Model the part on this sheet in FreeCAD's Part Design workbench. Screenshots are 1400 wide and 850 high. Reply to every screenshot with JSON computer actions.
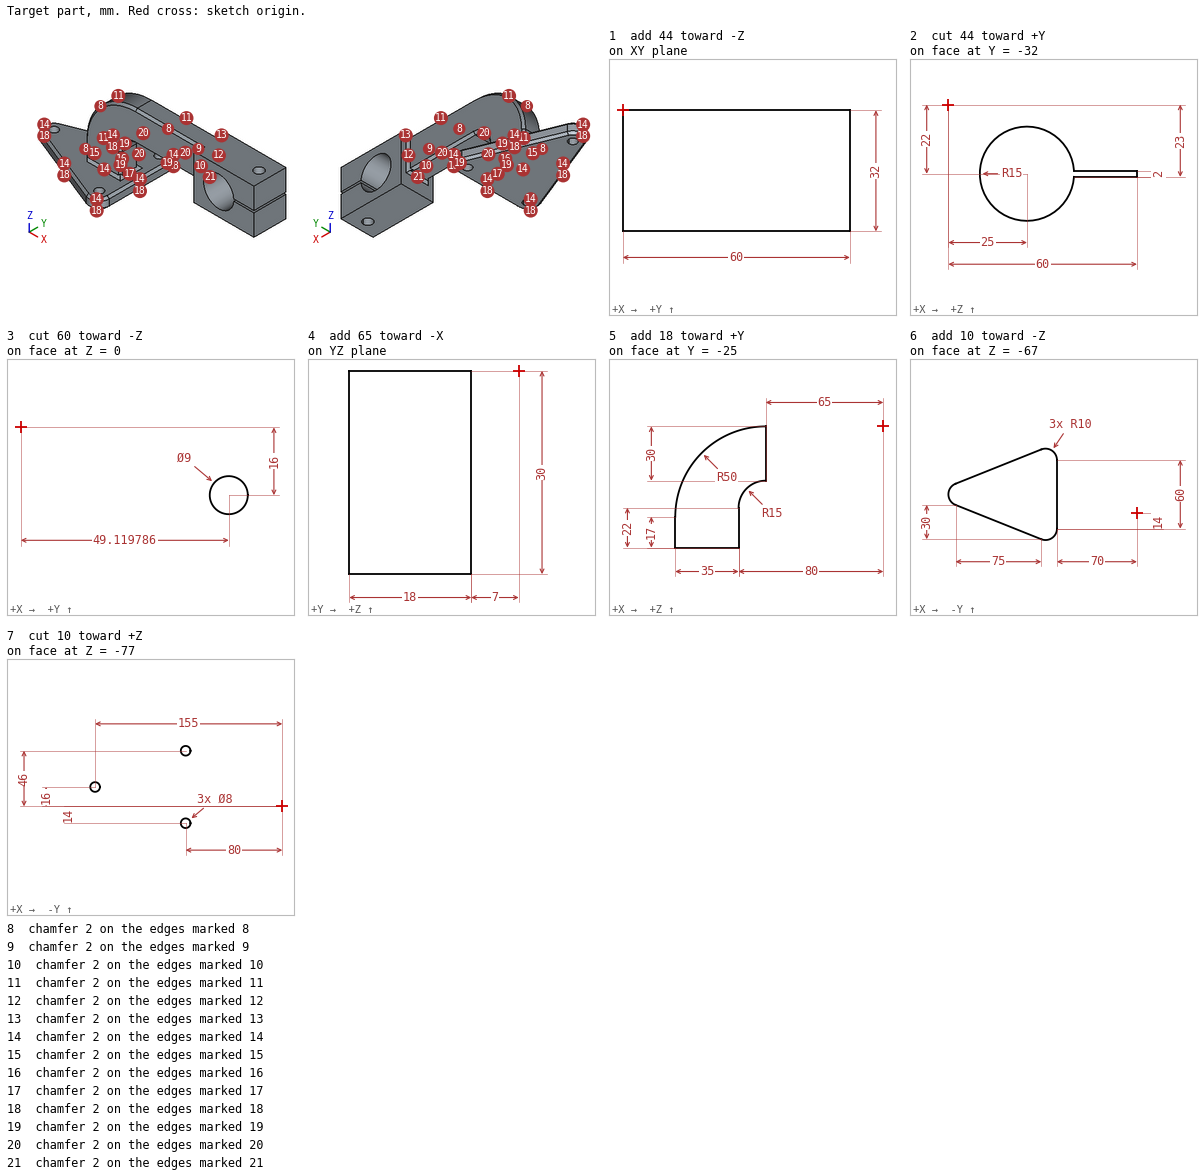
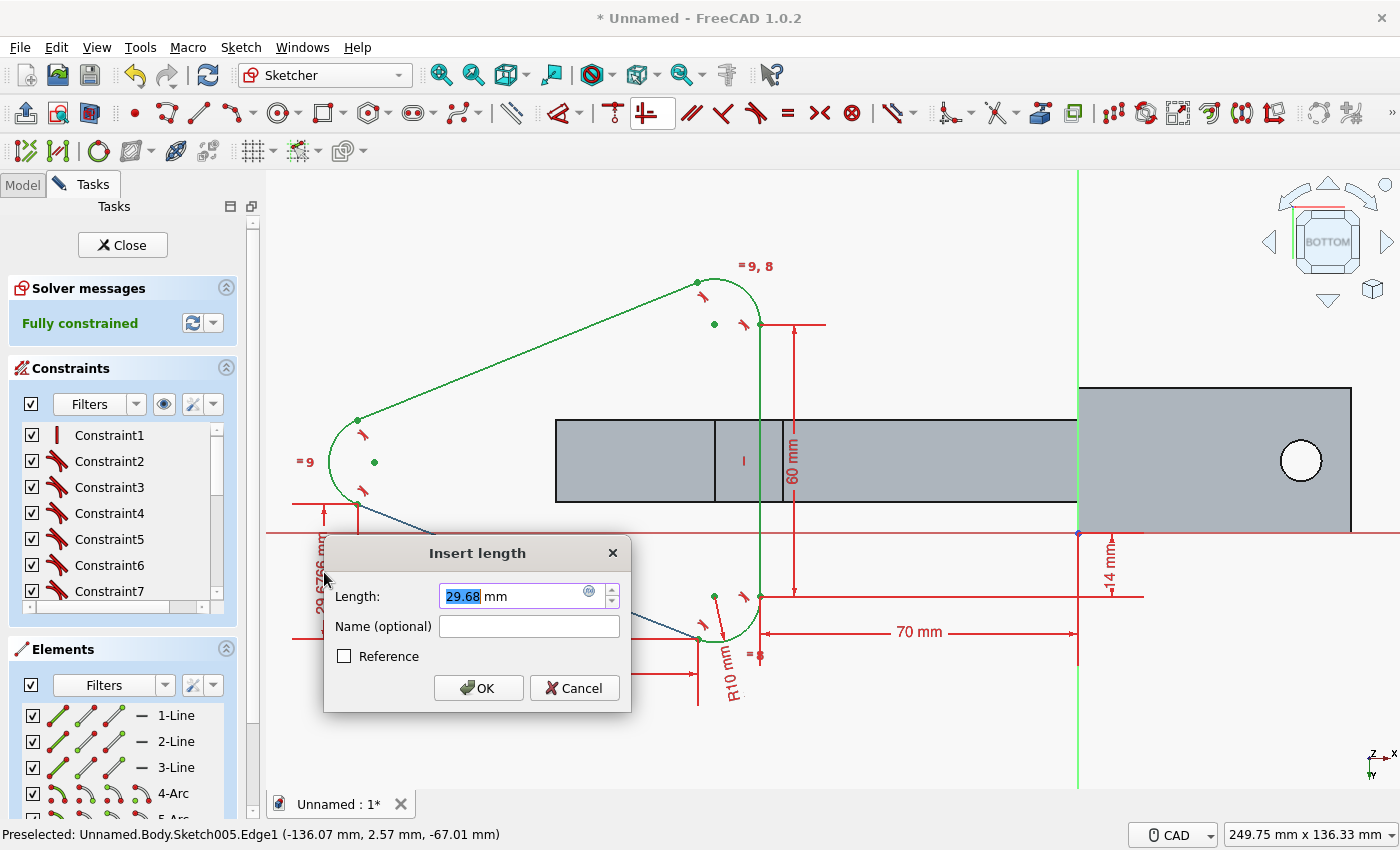
{"action": "type", "text": "30"}
{"action": "key", "text": "Return"}
{"action": "key", "text": "Escape"}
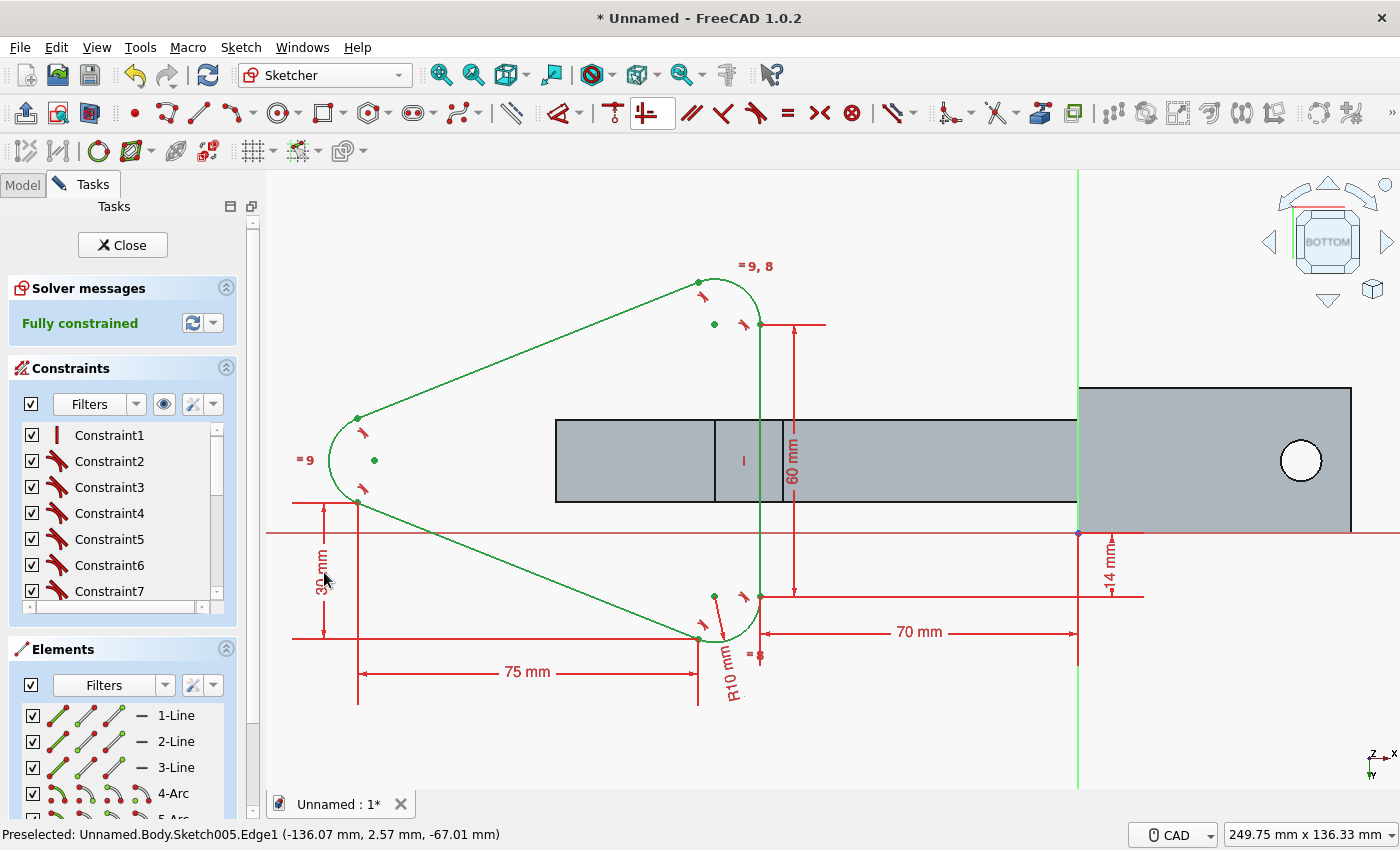
{"action": "left_click", "coordinate": [123, 245]}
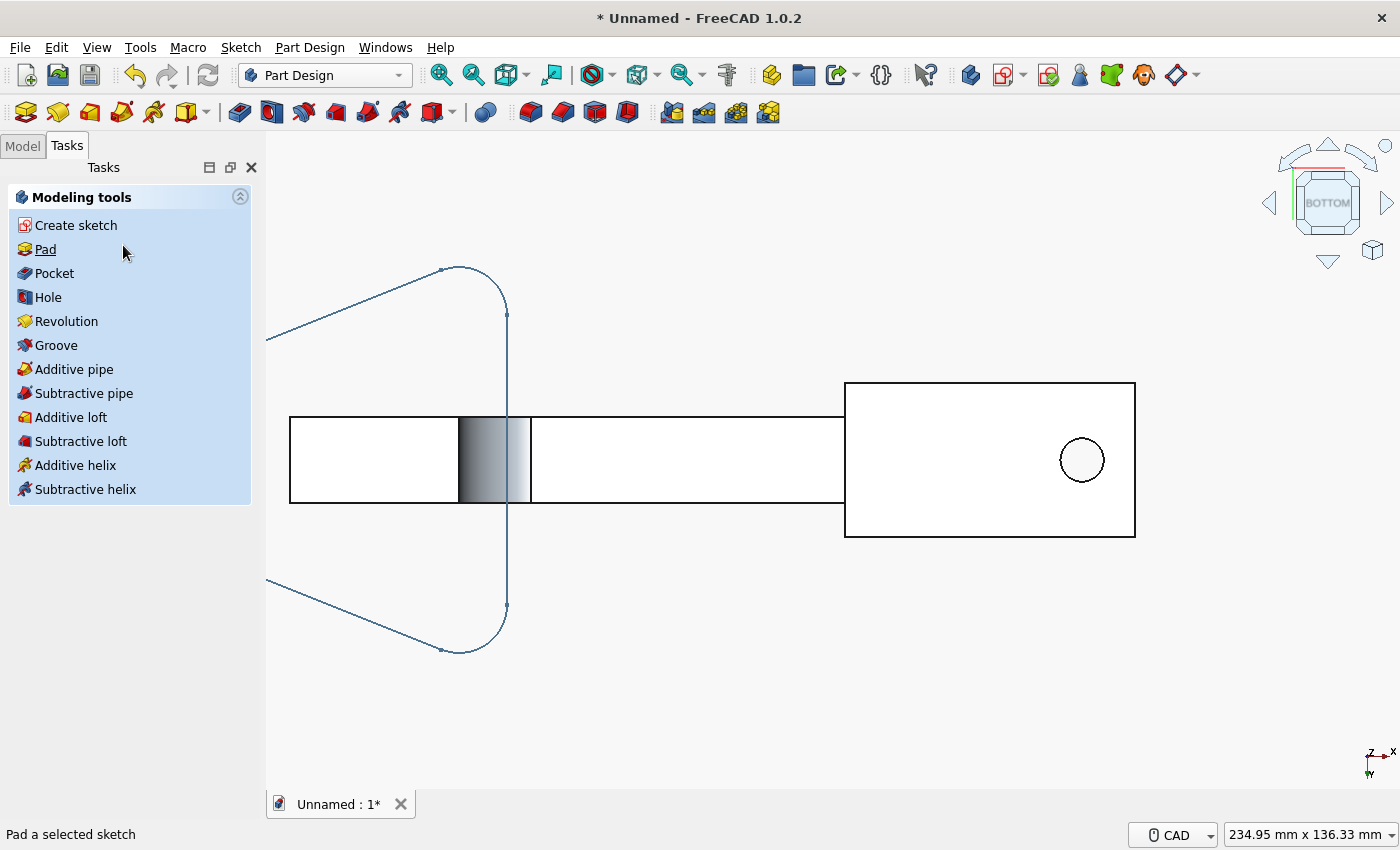
{"action": "left_click", "coordinate": [26, 112]}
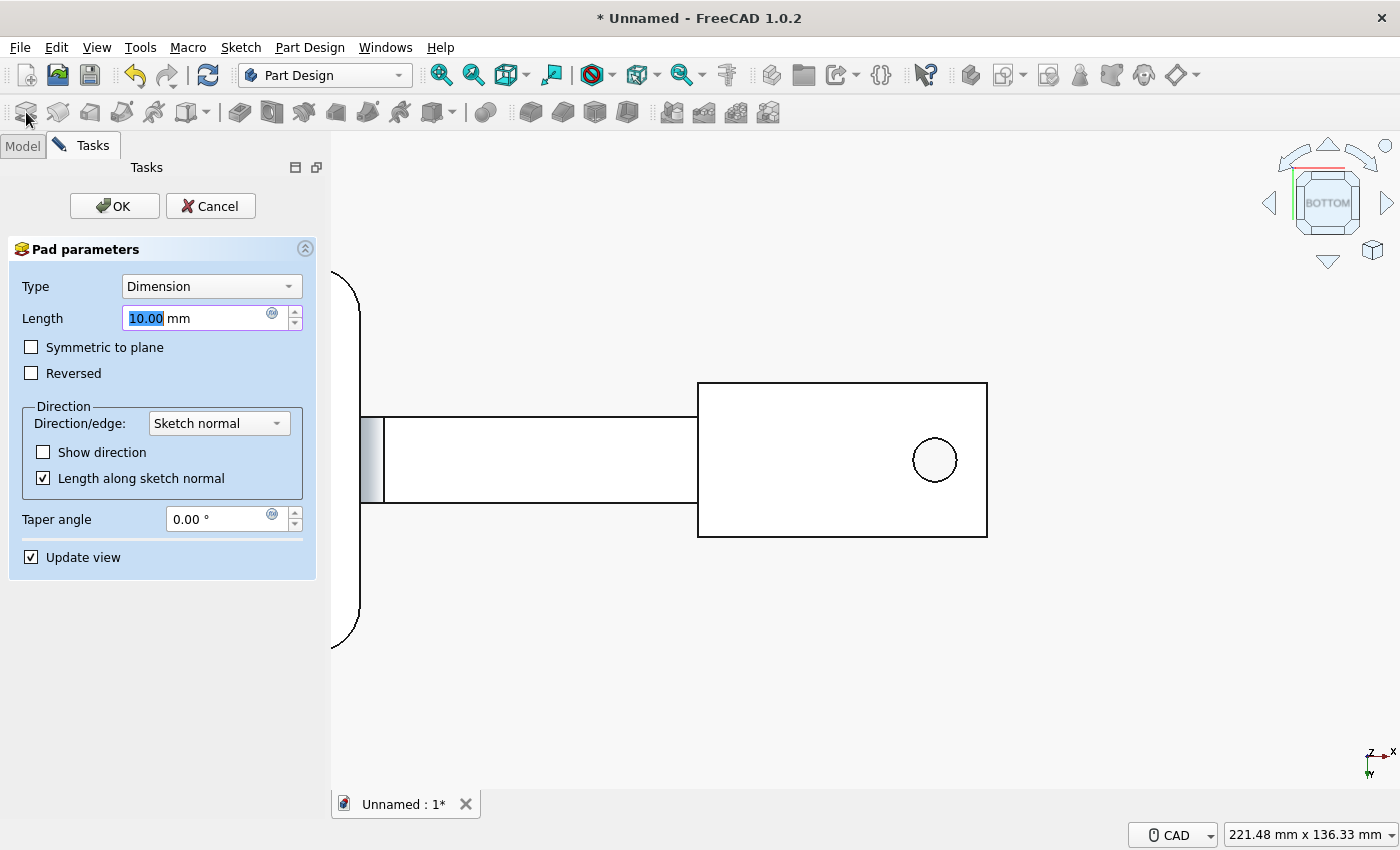
{"action": "type", "text": "10"}
{"action": "key", "text": "Tab"}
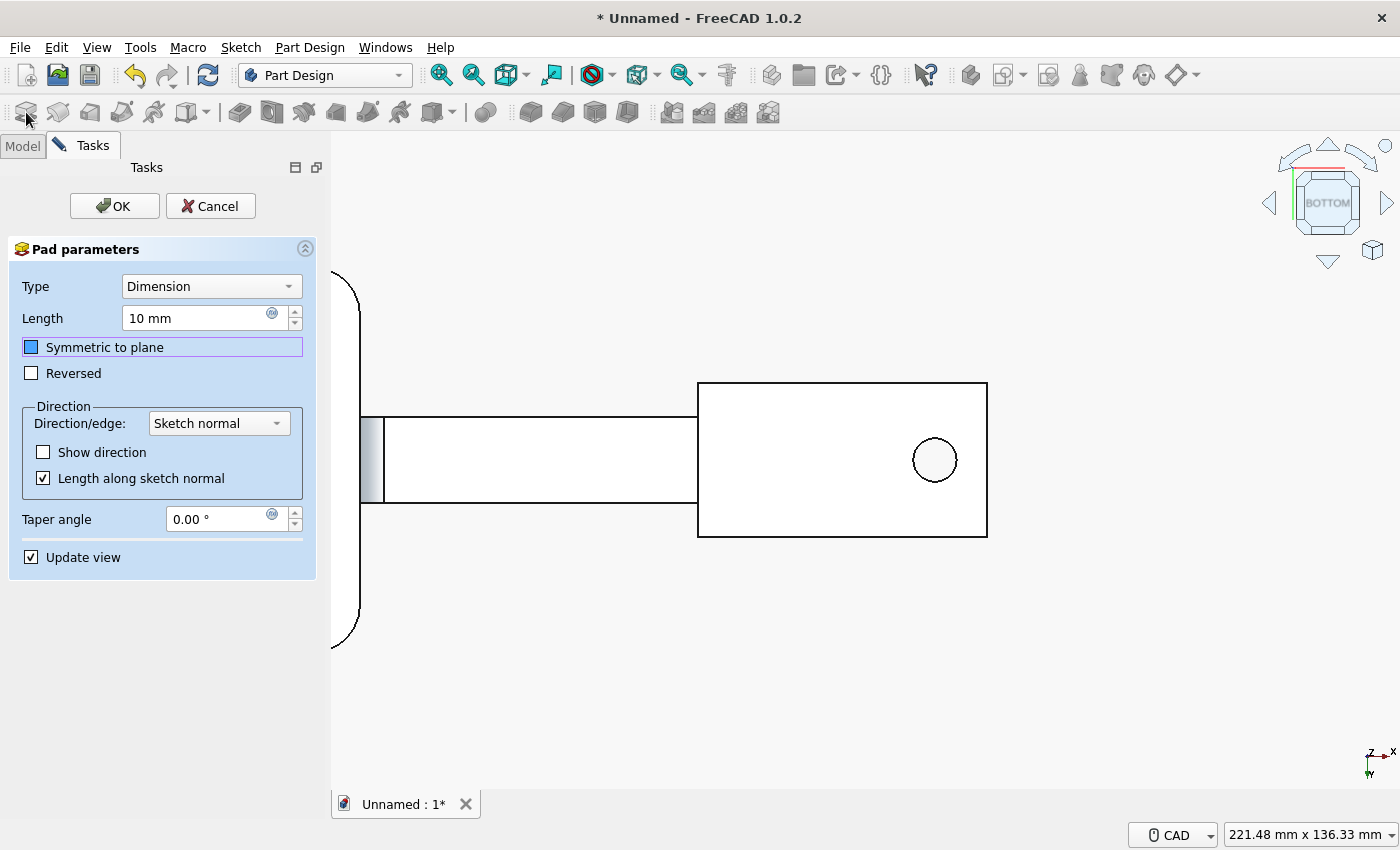
{"action": "left_click", "coordinate": [115, 206]}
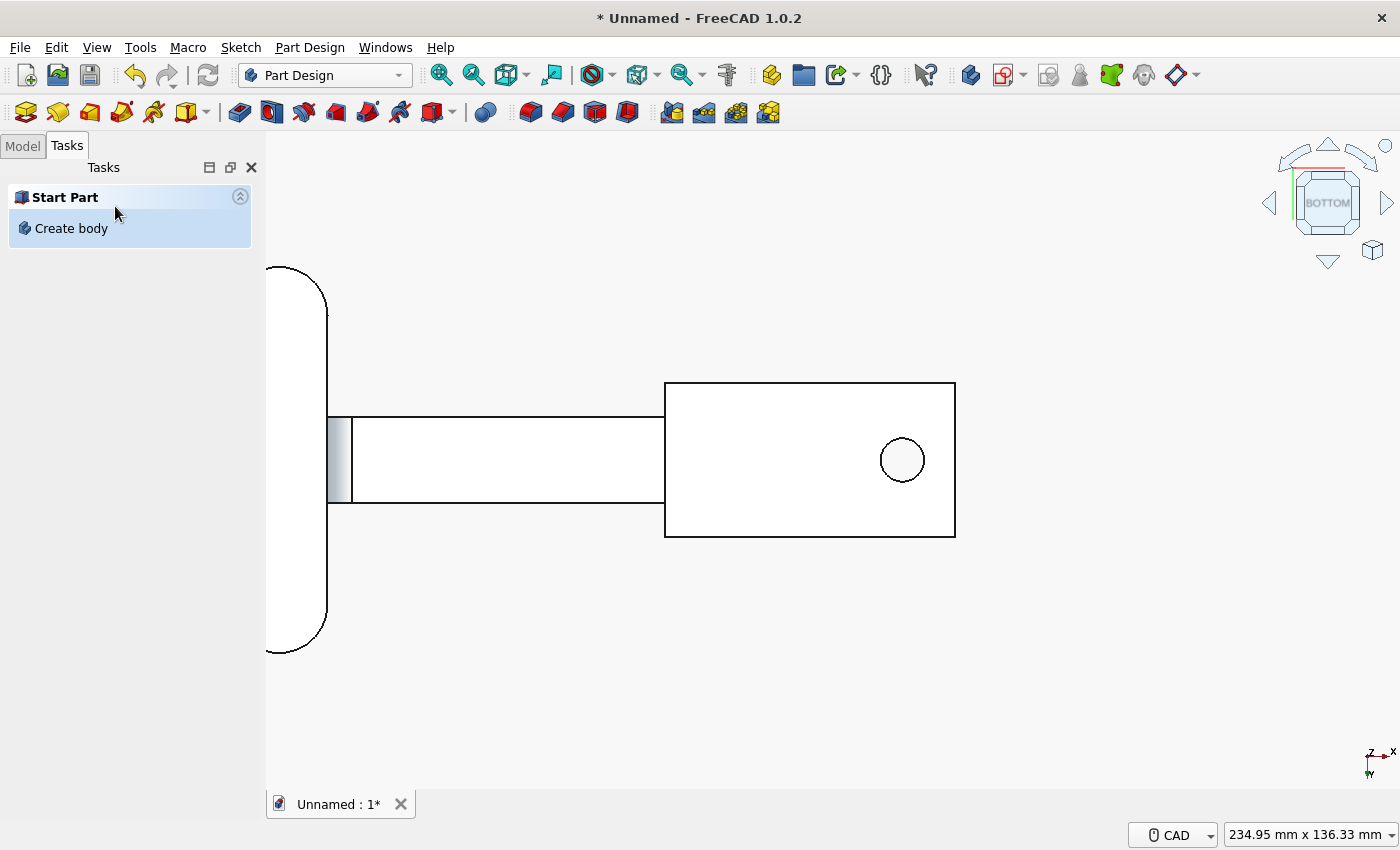
{"action": "left_click", "coordinate": [442, 76]}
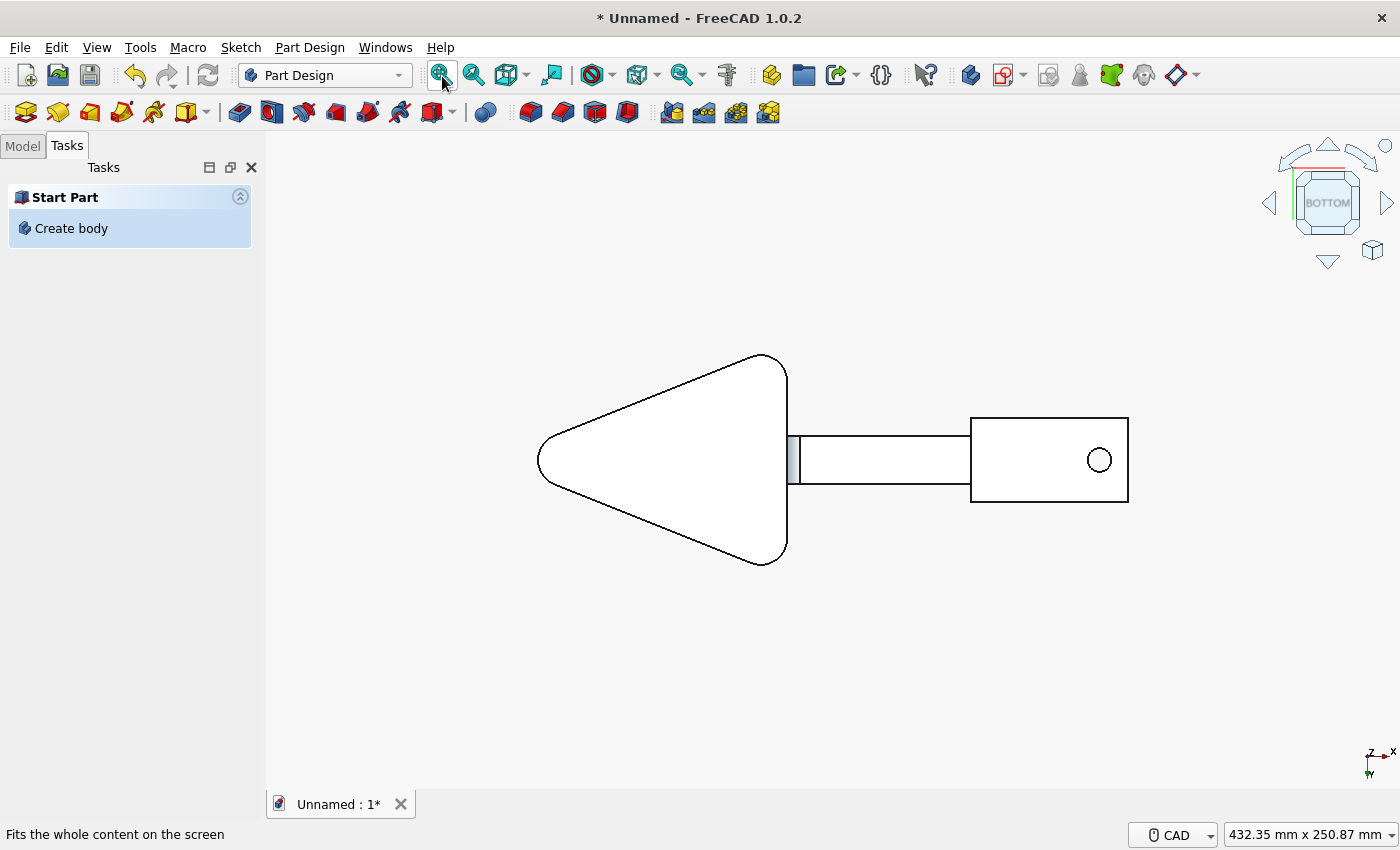
{"action": "left_click", "coordinate": [698, 459]}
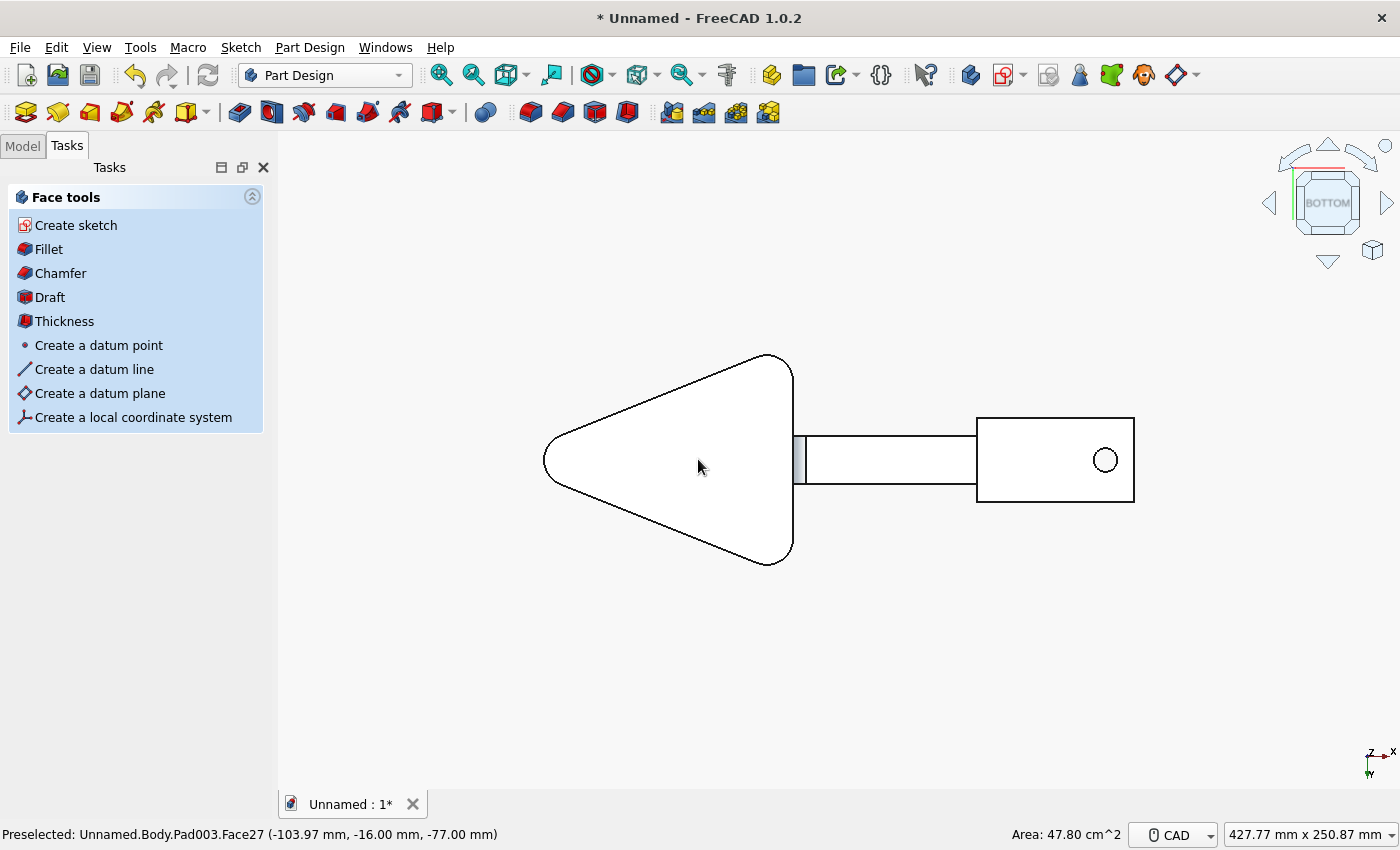
{"action": "left_click", "coordinate": [1004, 76]}